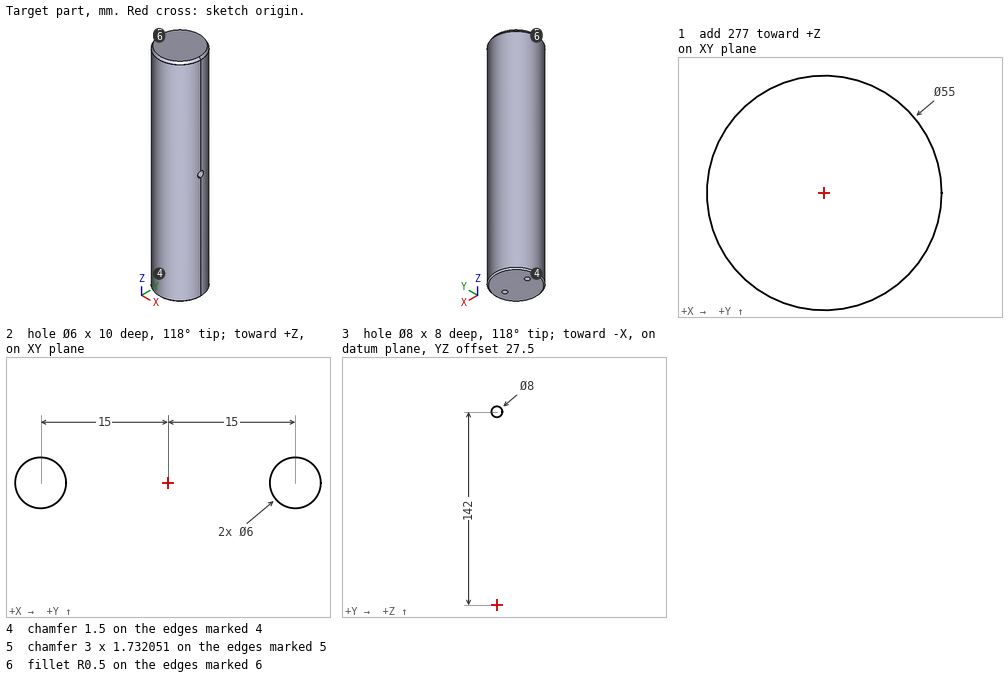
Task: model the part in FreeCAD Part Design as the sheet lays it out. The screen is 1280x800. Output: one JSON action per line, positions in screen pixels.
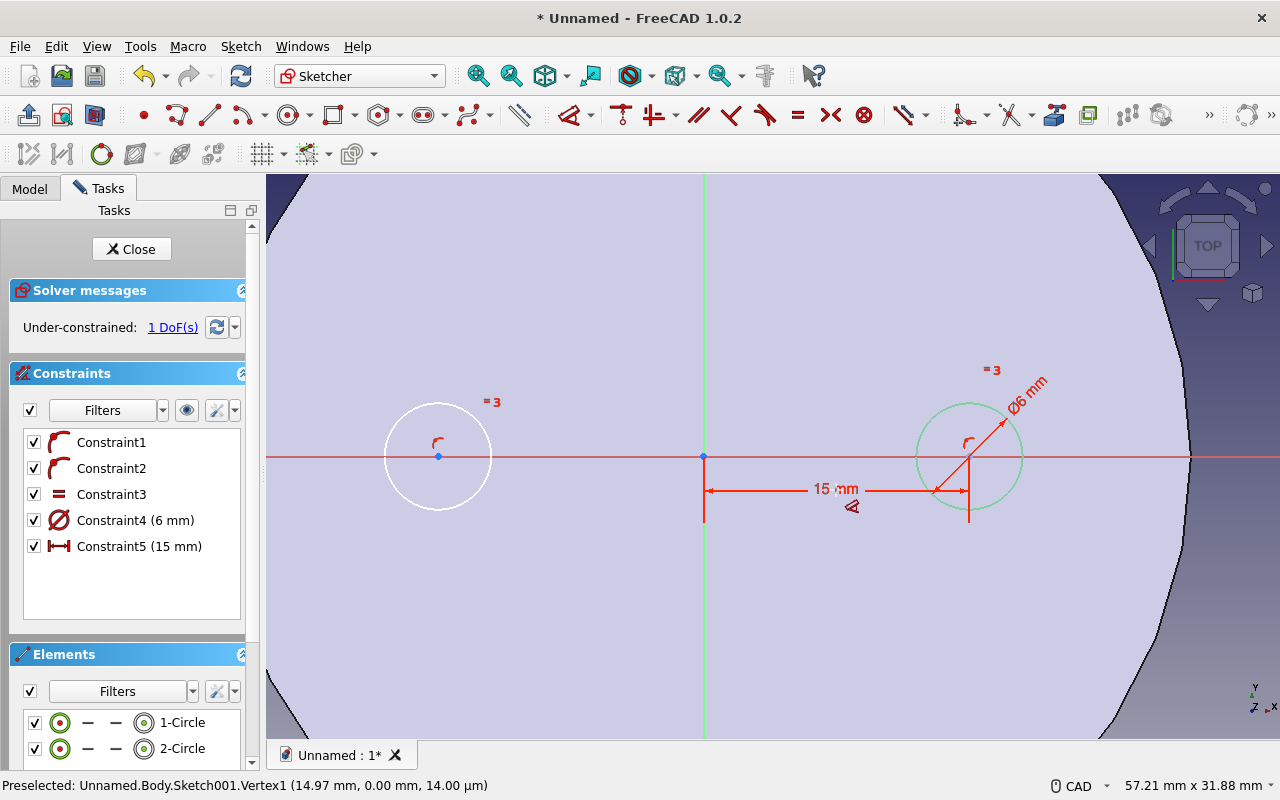
{"action": "left_click", "coordinate": [438, 456]}
{"action": "left_click", "coordinate": [571, 490]}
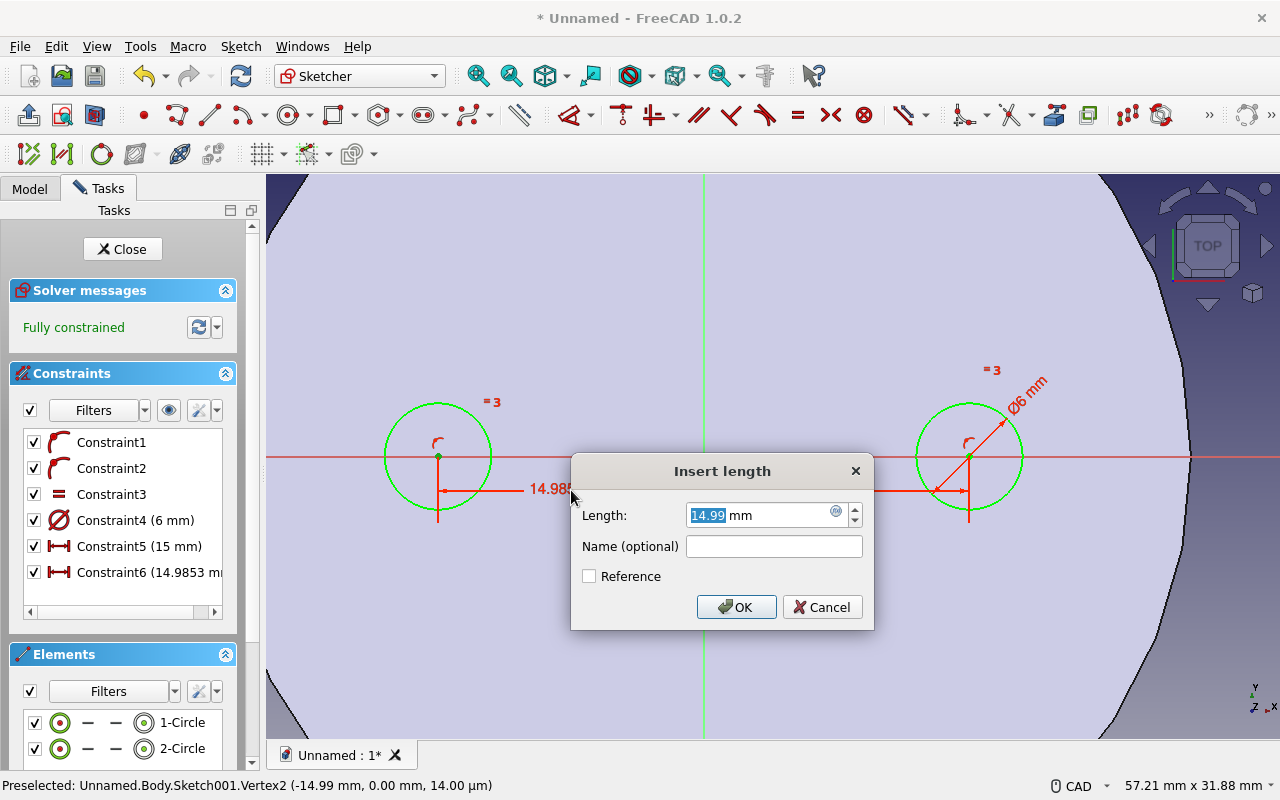
{"action": "type", "text": "15"}
{"action": "key", "text": "Return"}
{"action": "key", "text": "Escape"}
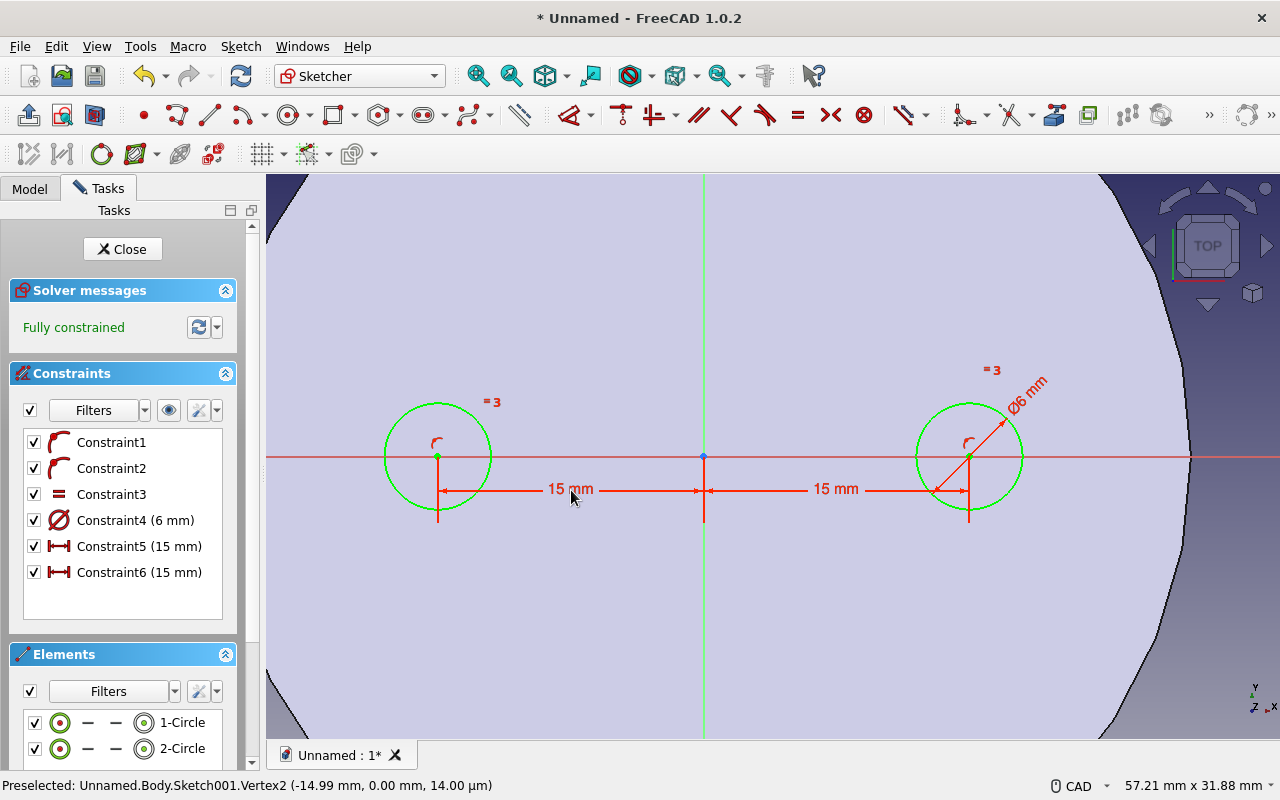
{"action": "left_click", "coordinate": [123, 249]}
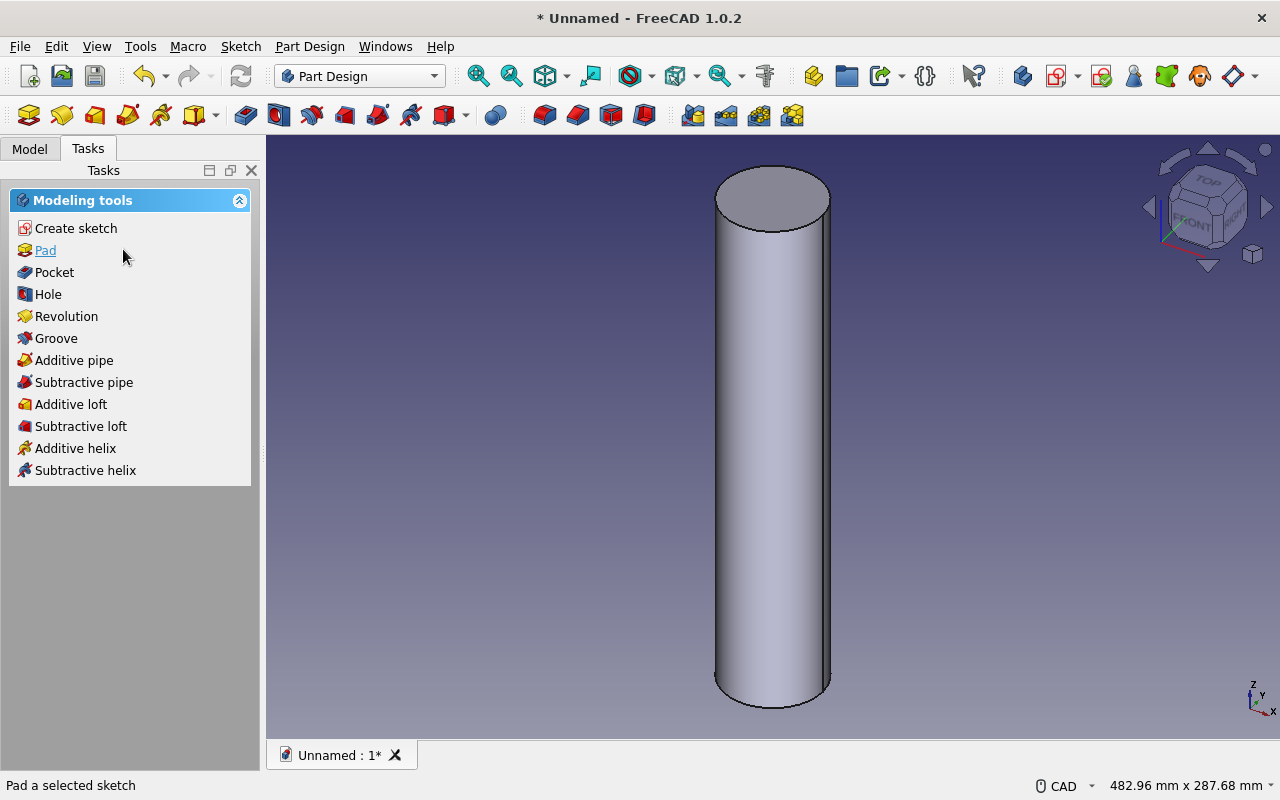
{"action": "left_click", "coordinate": [279, 116]}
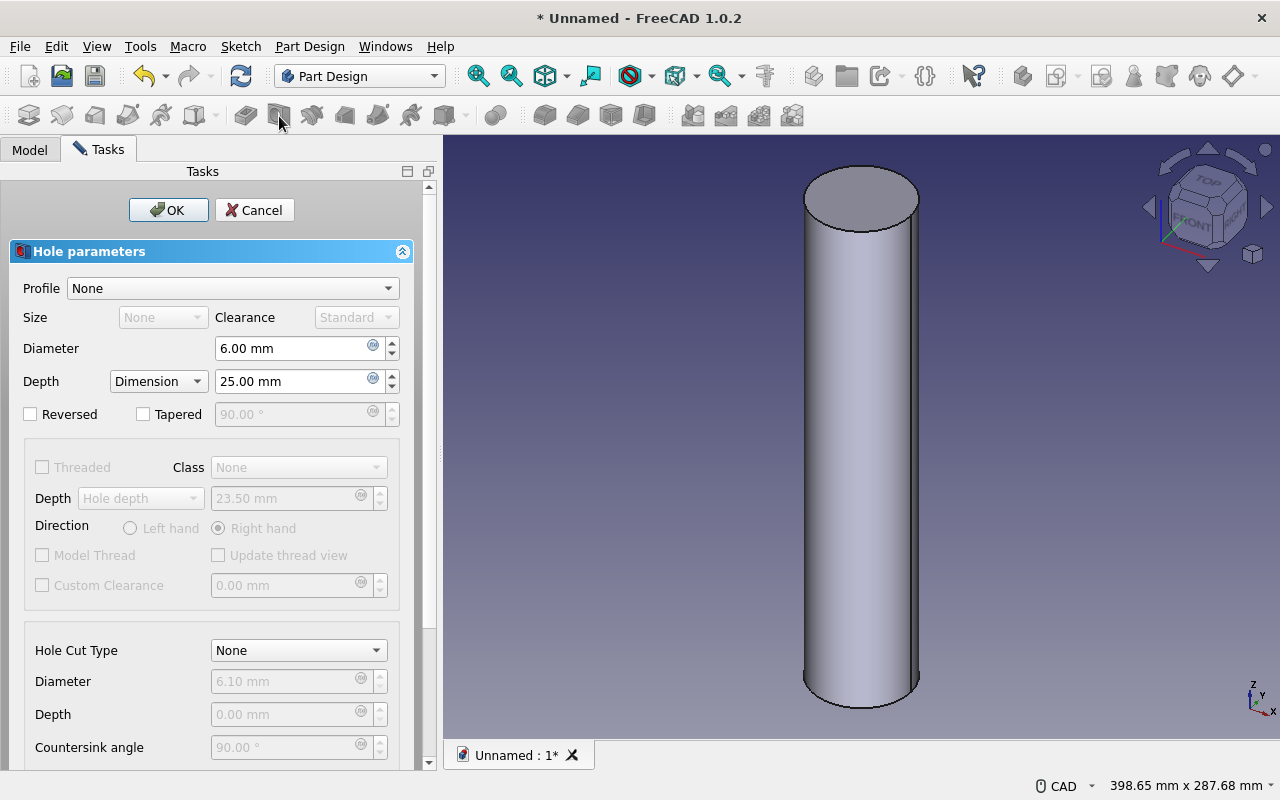
{"action": "triple_click", "coordinate": [300, 348]}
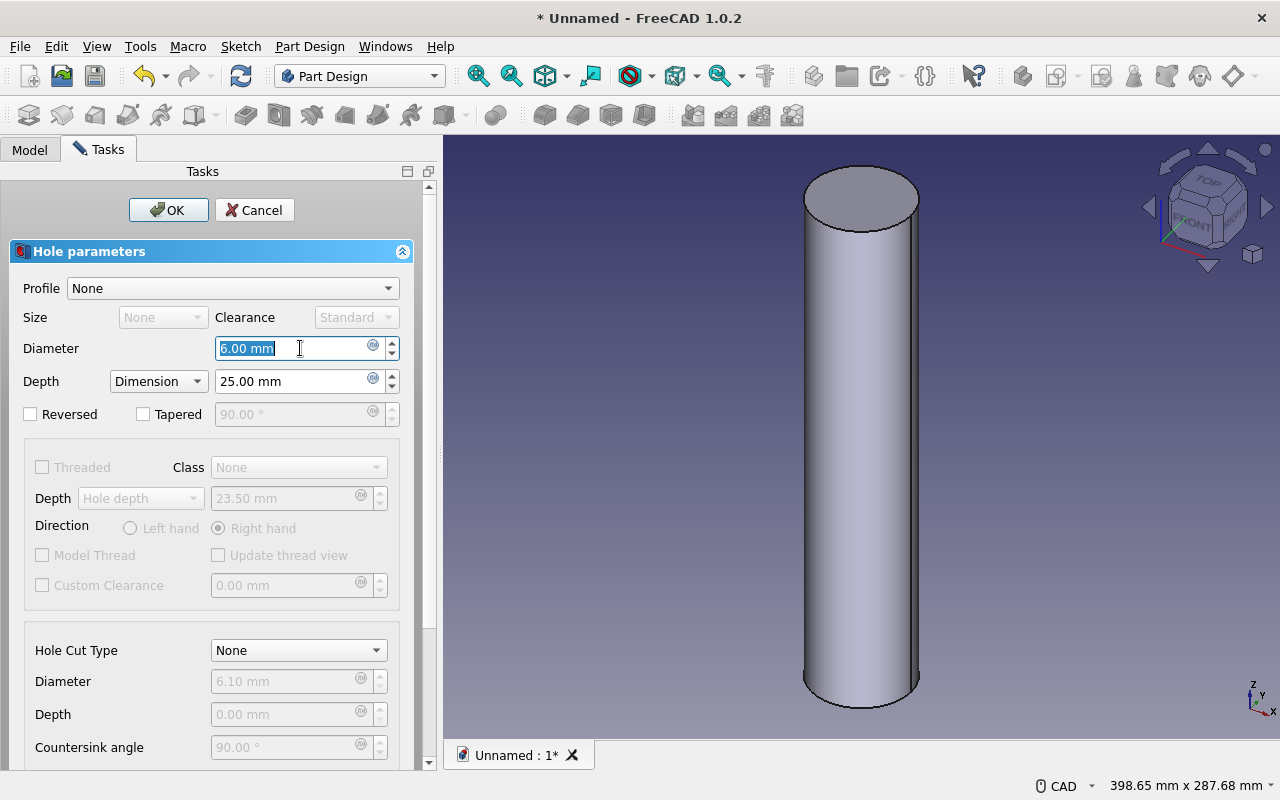
{"action": "type", "text": "6"}
{"action": "key", "text": "Tab"}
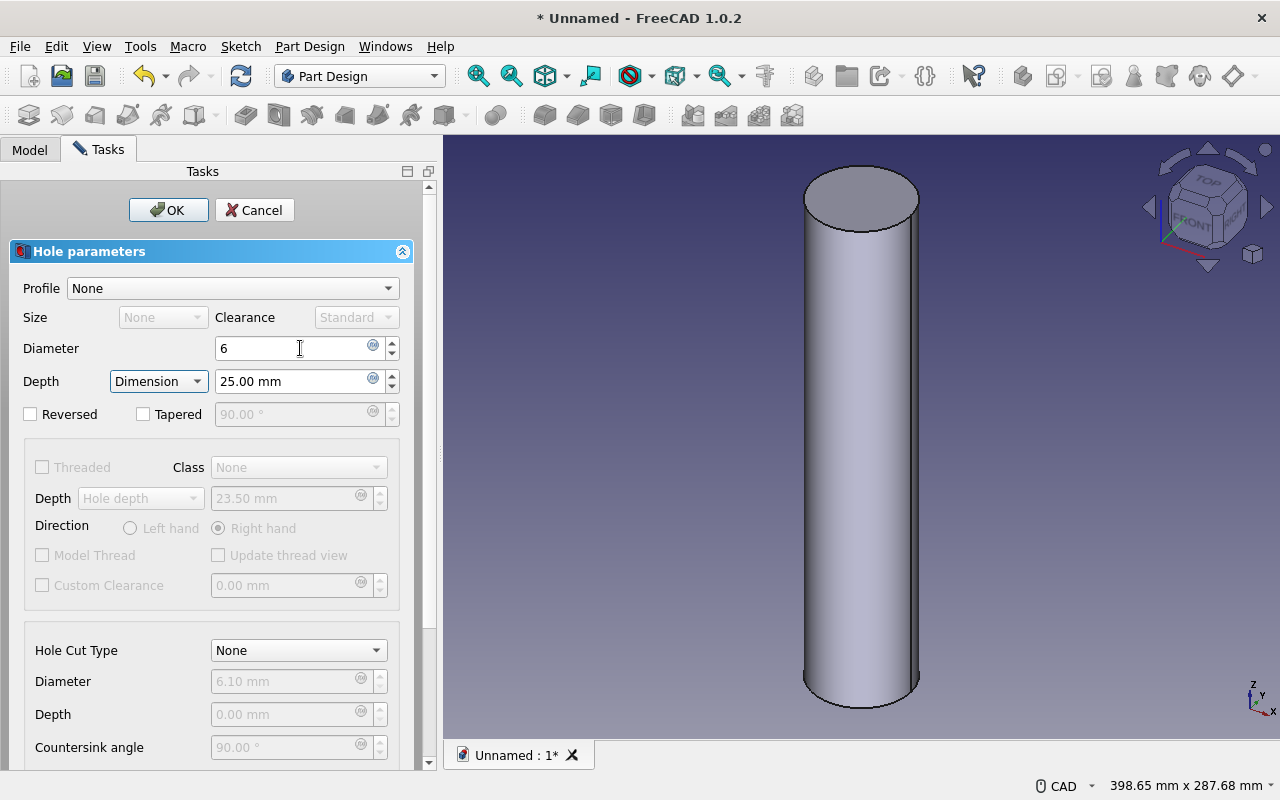
{"action": "triple_click", "coordinate": [300, 382]}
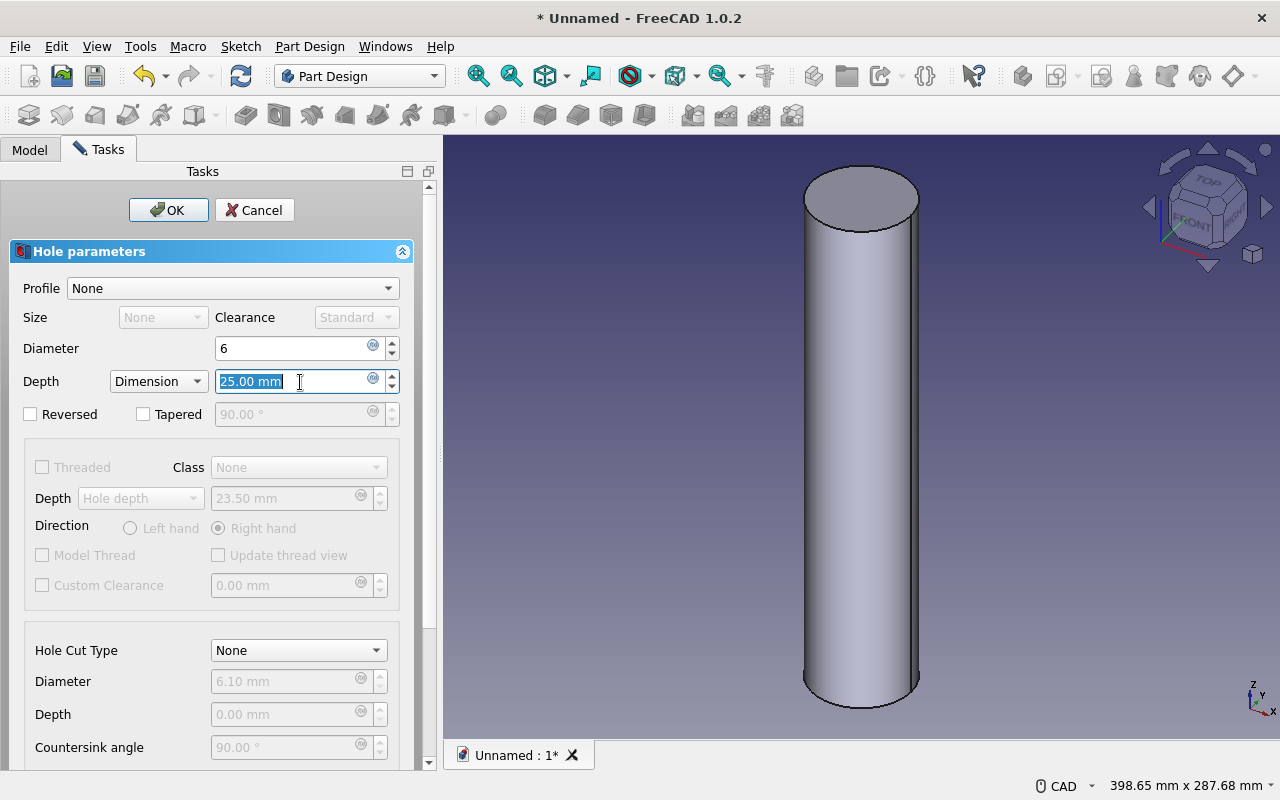
{"action": "type", "text": "10"}
{"action": "key", "text": "Tab"}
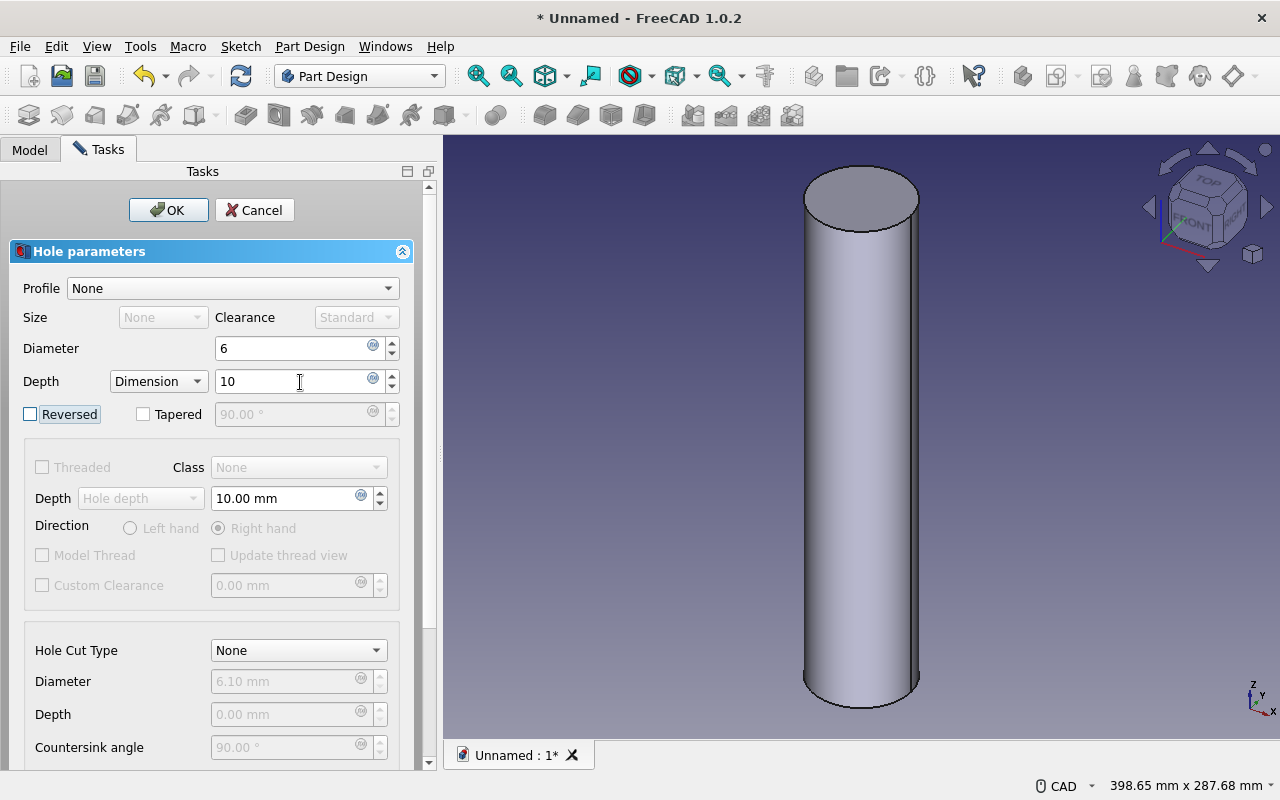
{"action": "left_click", "coordinate": [31, 414]}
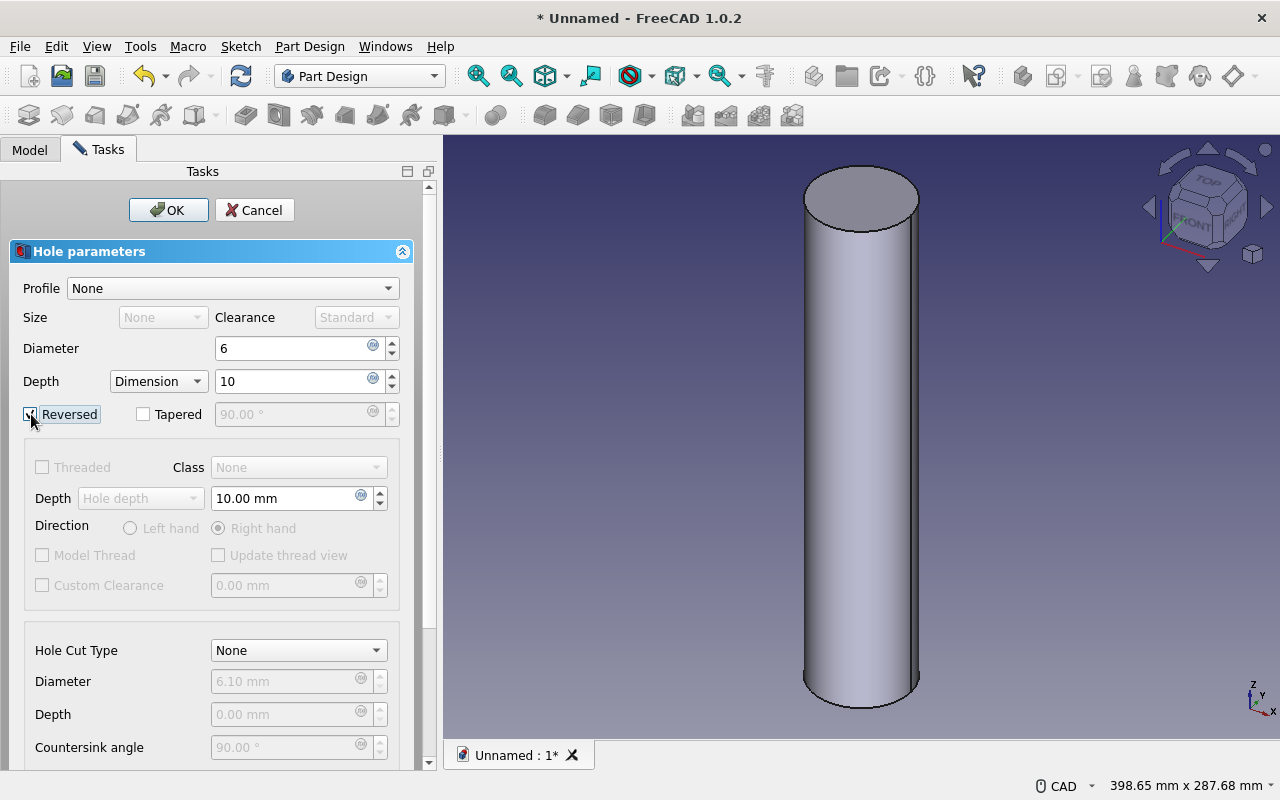
{"action": "left_click", "coordinate": [169, 210]}